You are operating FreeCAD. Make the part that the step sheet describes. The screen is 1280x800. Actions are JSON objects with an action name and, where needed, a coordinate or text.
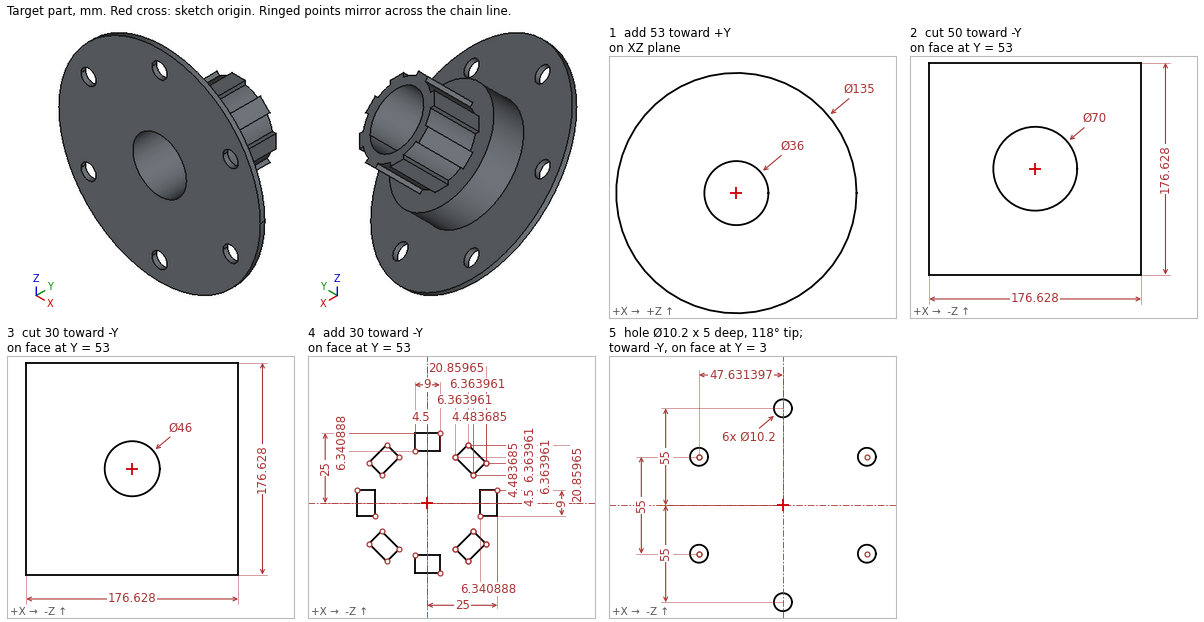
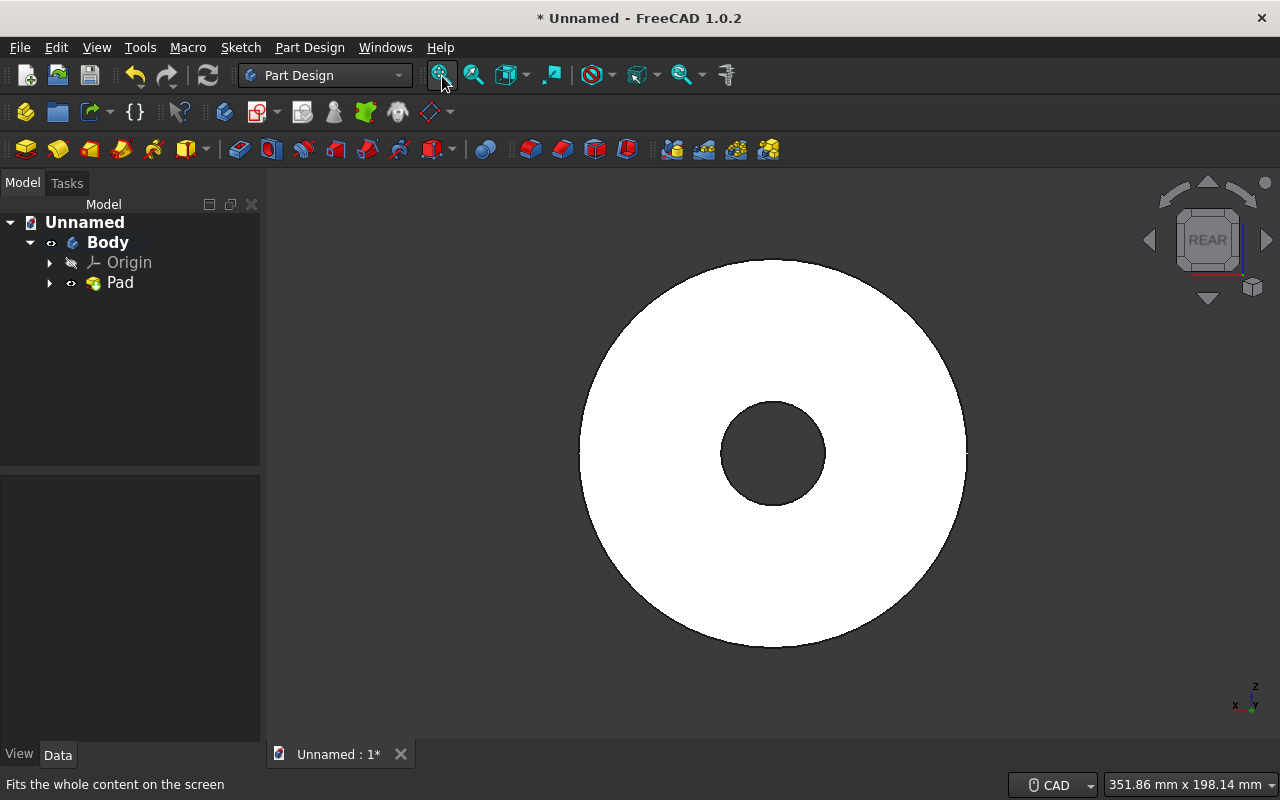
{"action": "left_click", "coordinate": [884, 508]}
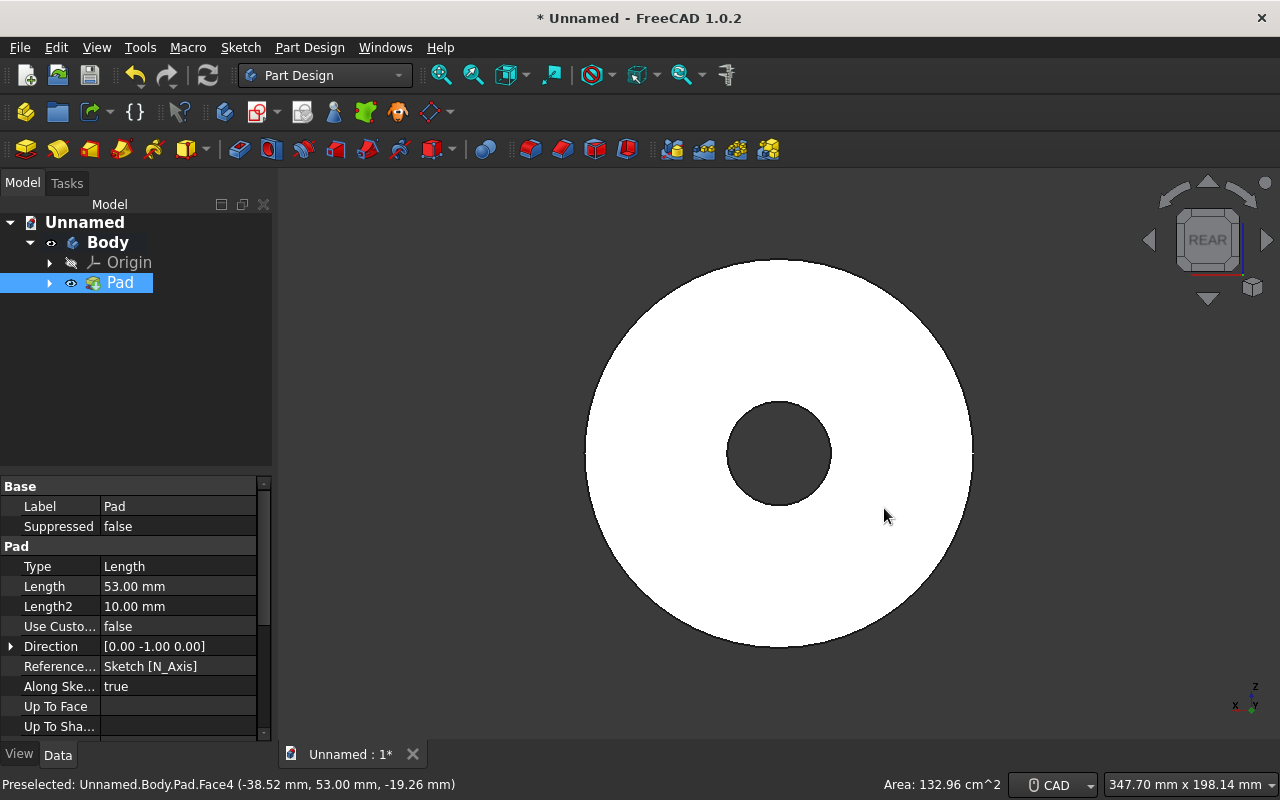
{"action": "left_click", "coordinate": [258, 112]}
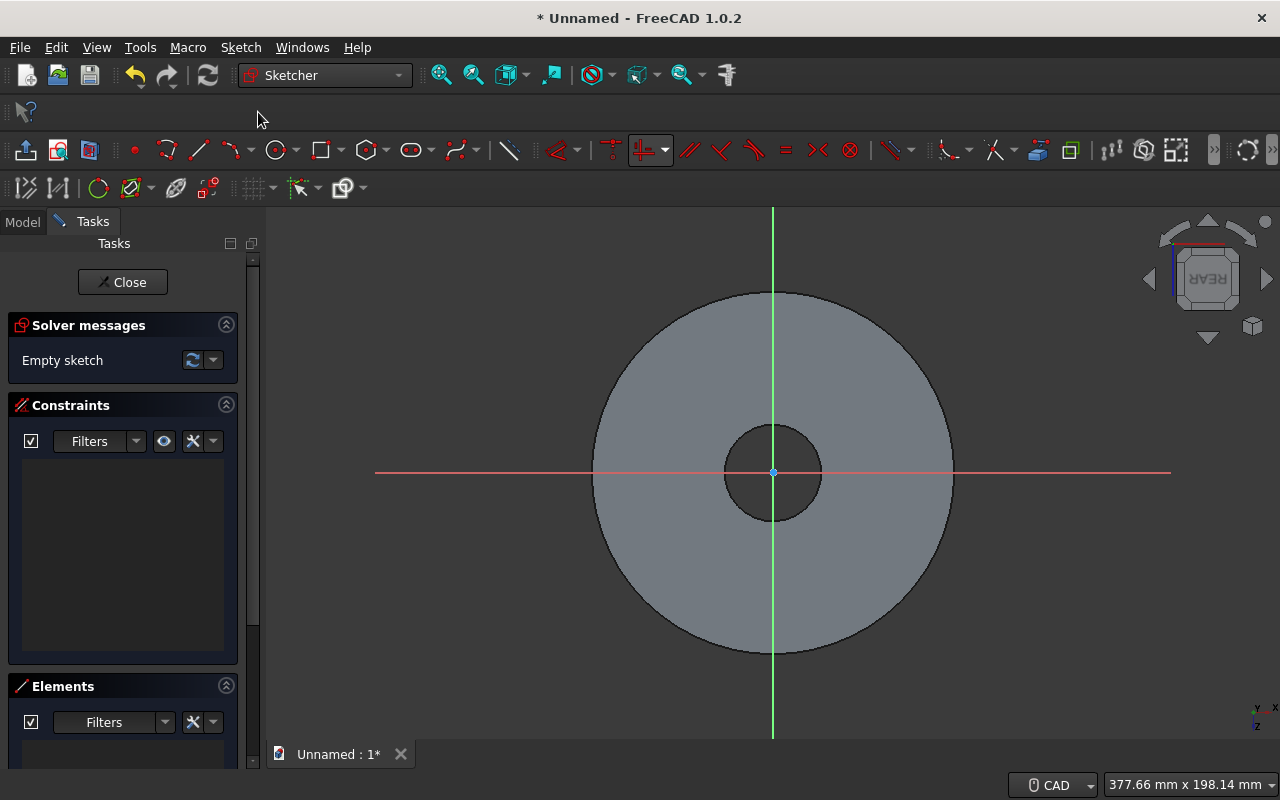
{"action": "scroll", "coordinate": [565, 473], "scroll_direction": "down", "scroll_amount": 2}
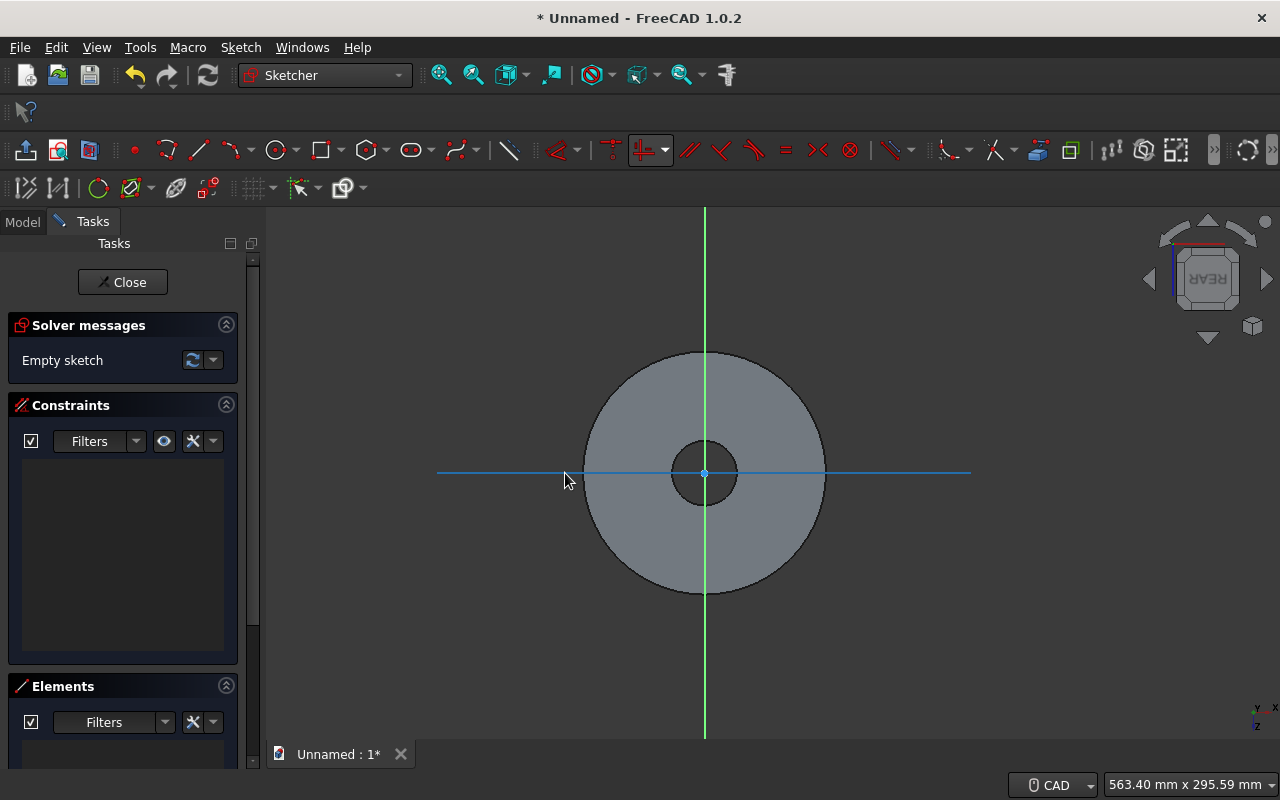
{"action": "left_click", "coordinate": [344, 150]}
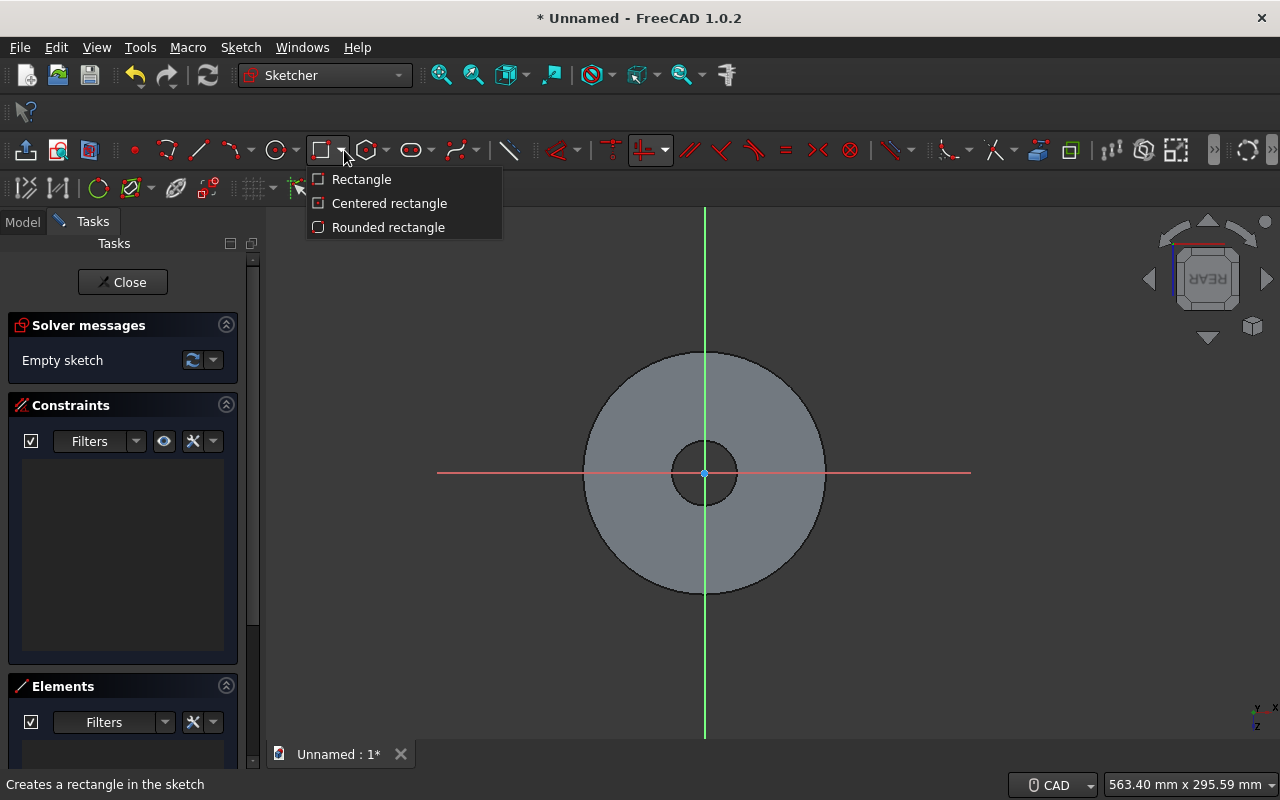
{"action": "left_click", "coordinate": [404, 203]}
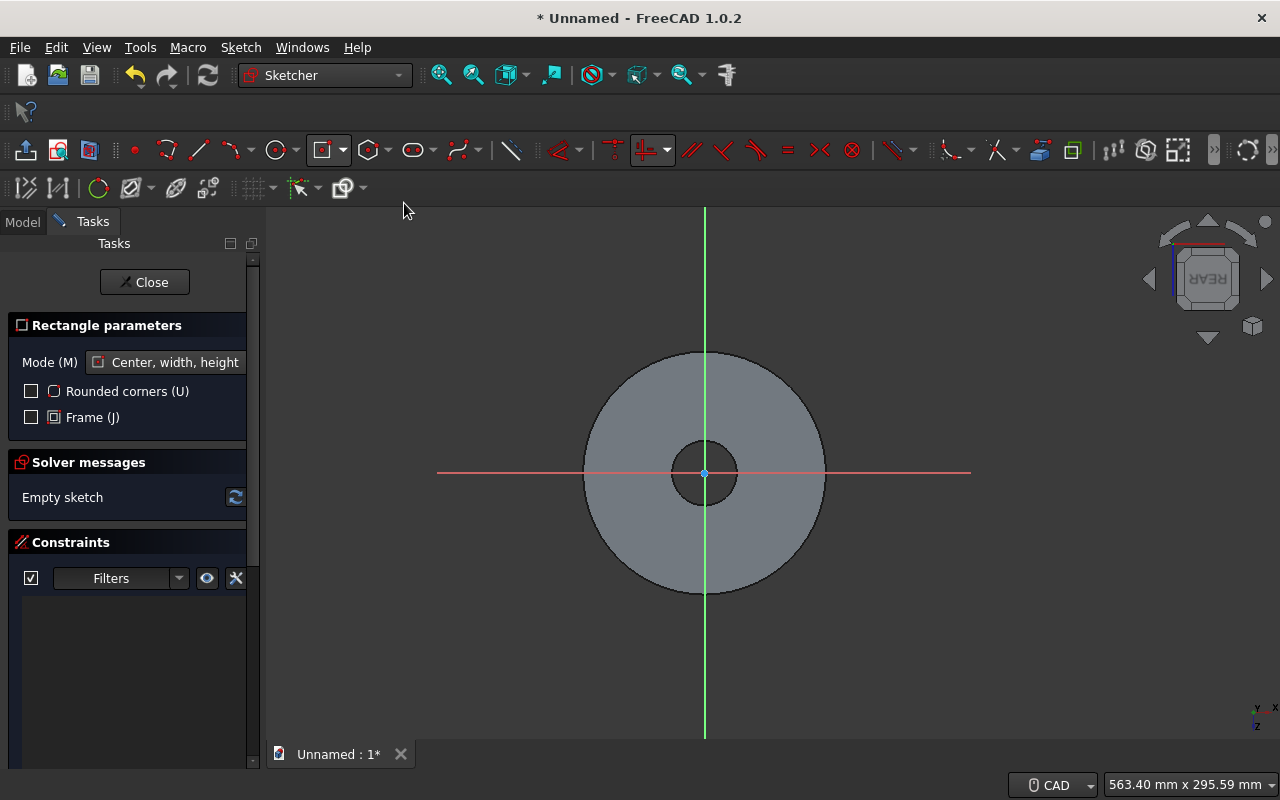
{"action": "left_click", "coordinate": [705, 473]}
{"action": "left_click", "coordinate": [863, 314]}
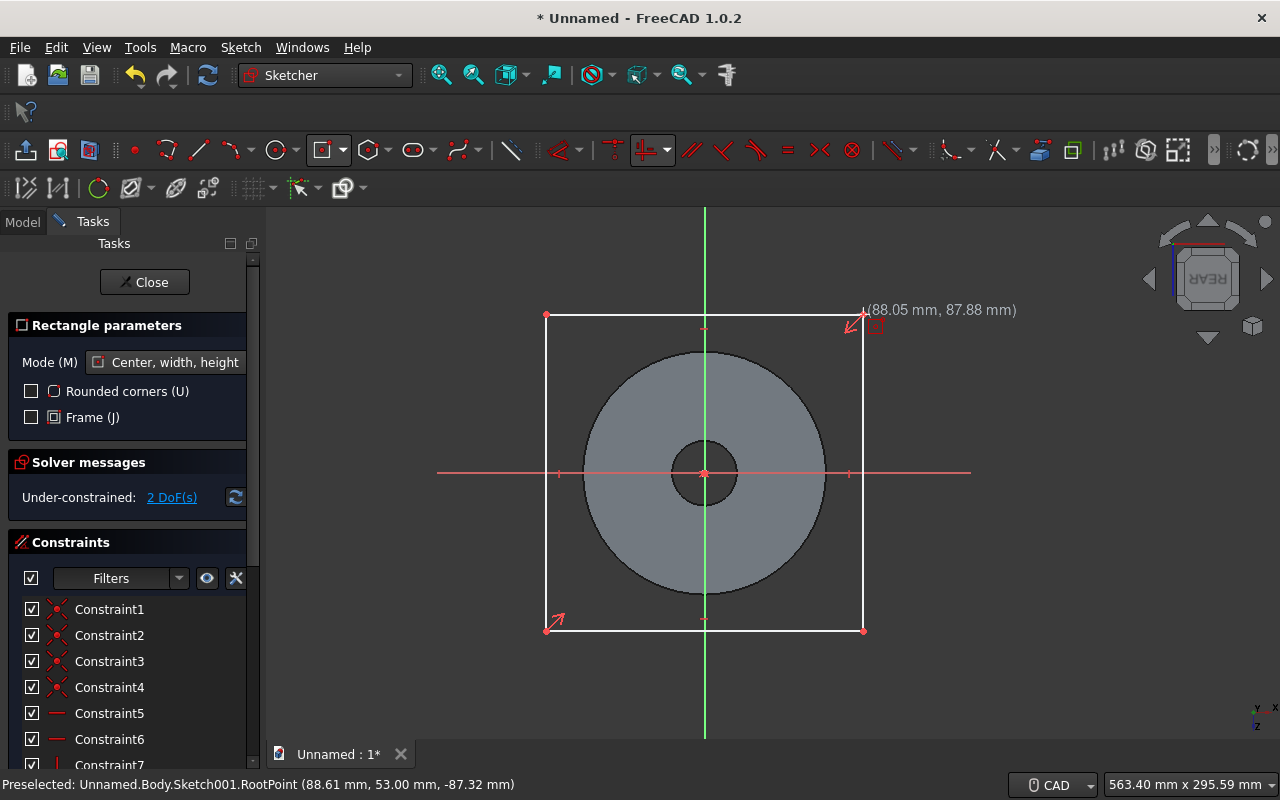
{"action": "left_click", "coordinate": [276, 150]}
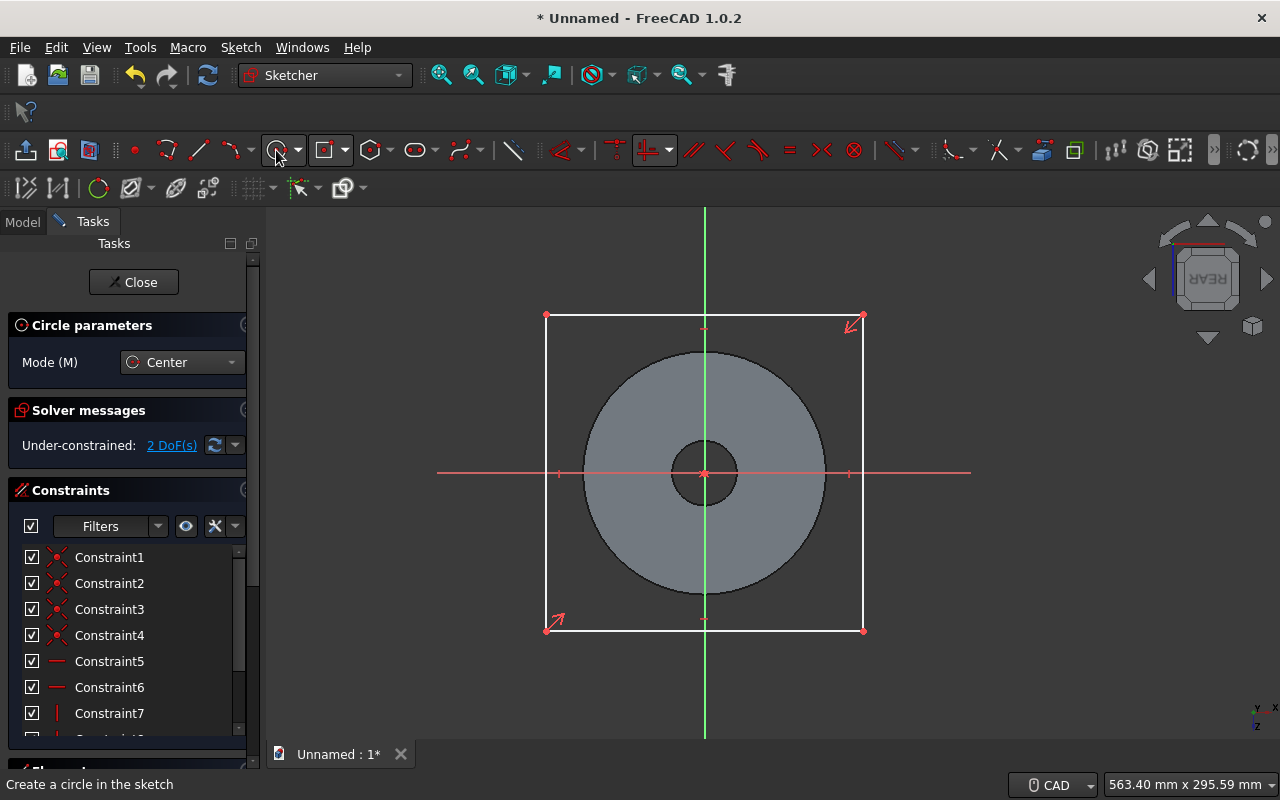
{"action": "left_click", "coordinate": [705, 473]}
{"action": "left_click", "coordinate": [749, 429]}
{"action": "key", "text": "Escape"}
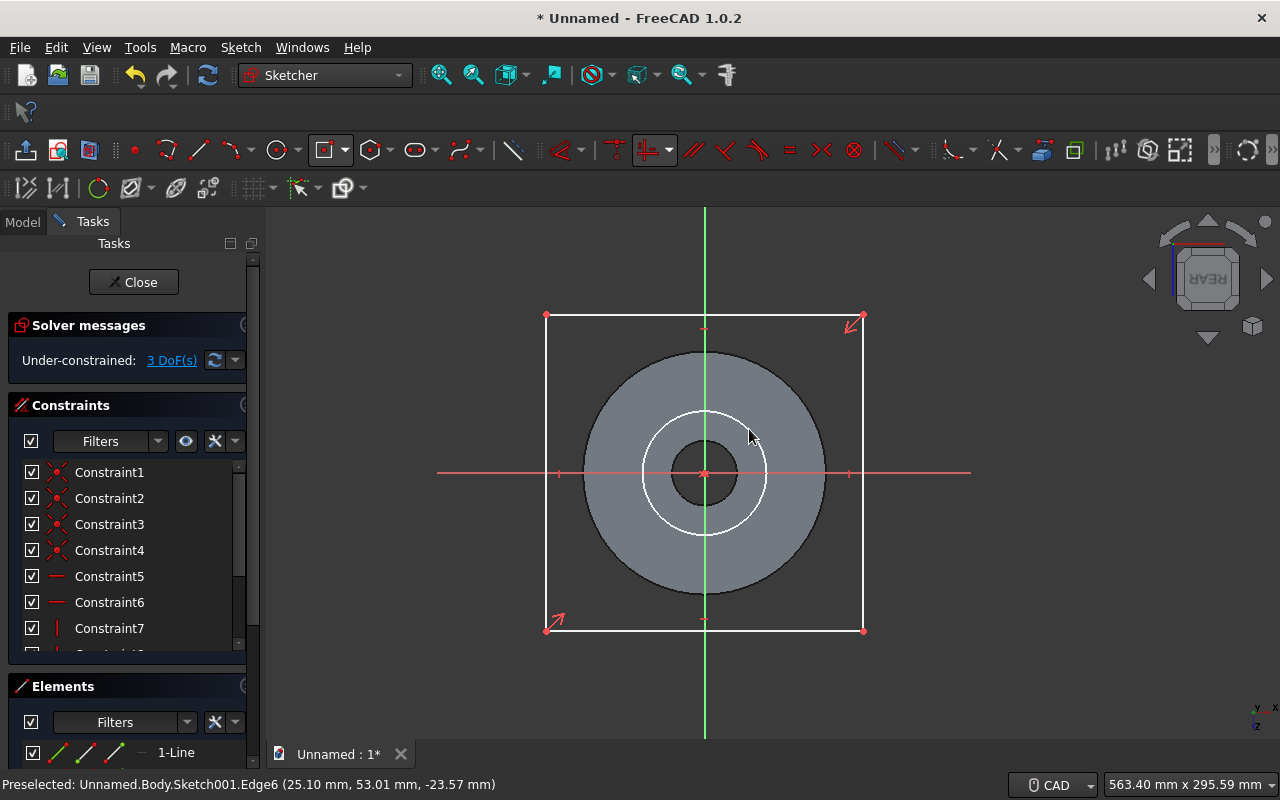
{"action": "left_click", "coordinate": [560, 150]}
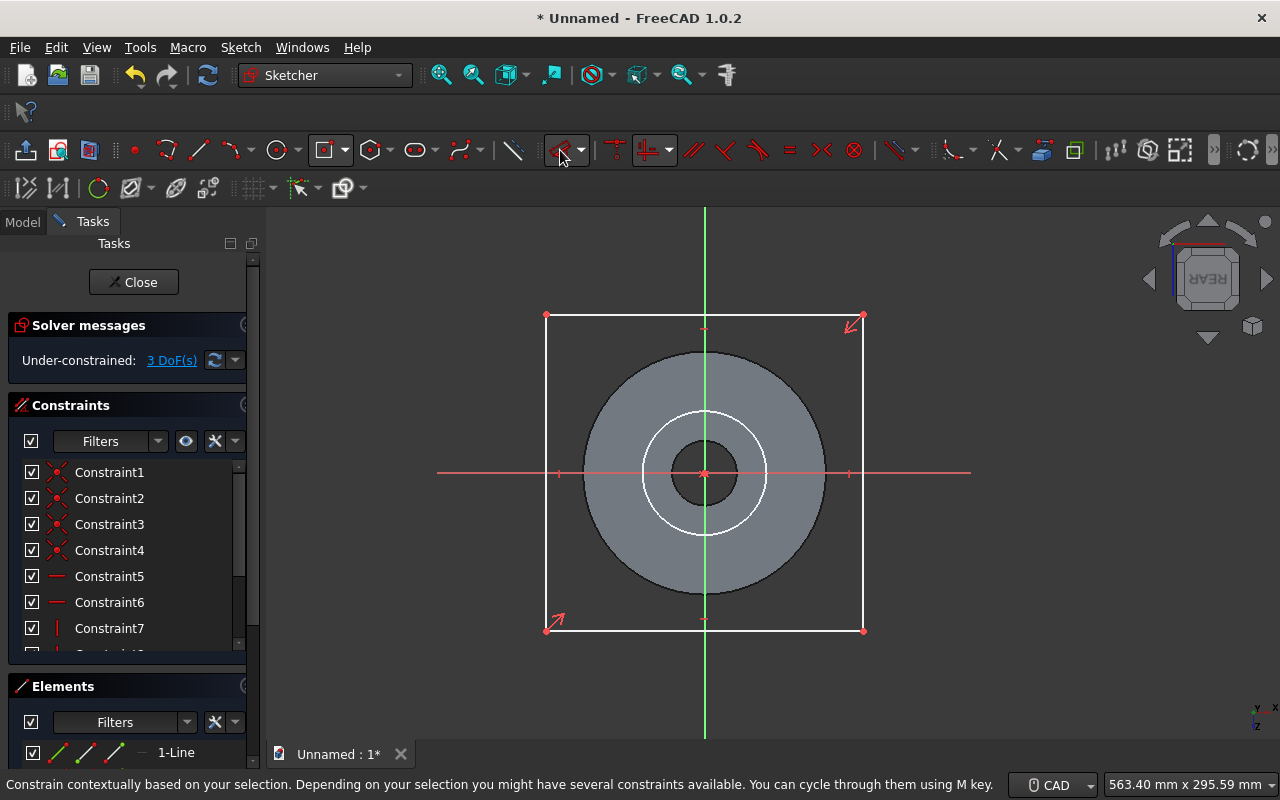
{"action": "left_click", "coordinate": [748, 429]}
{"action": "left_click", "coordinate": [770, 406]}